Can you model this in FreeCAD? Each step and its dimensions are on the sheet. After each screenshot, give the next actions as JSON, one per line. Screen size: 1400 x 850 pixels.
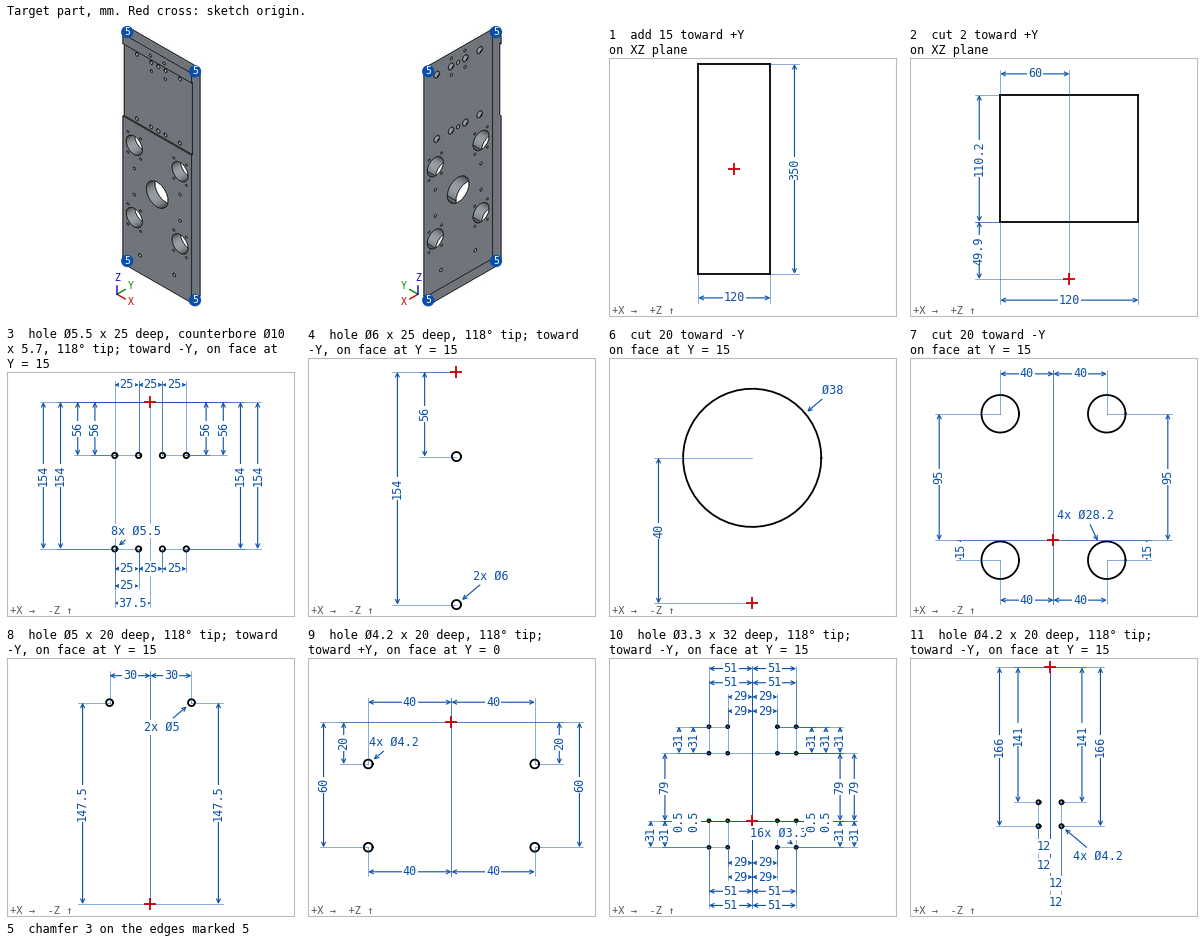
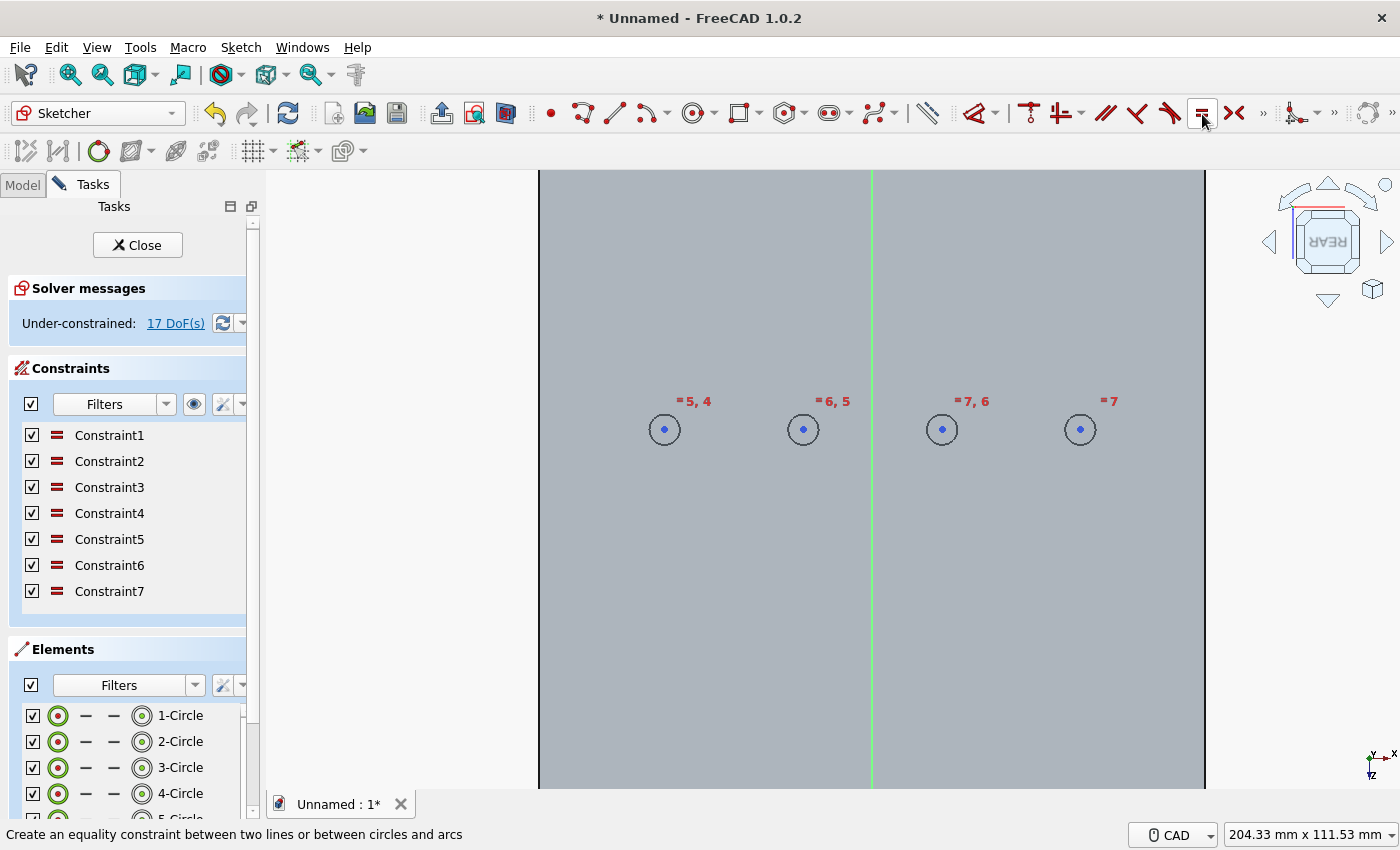
{"action": "scroll", "coordinate": [676, 419], "scroll_direction": "down", "scroll_amount": 4}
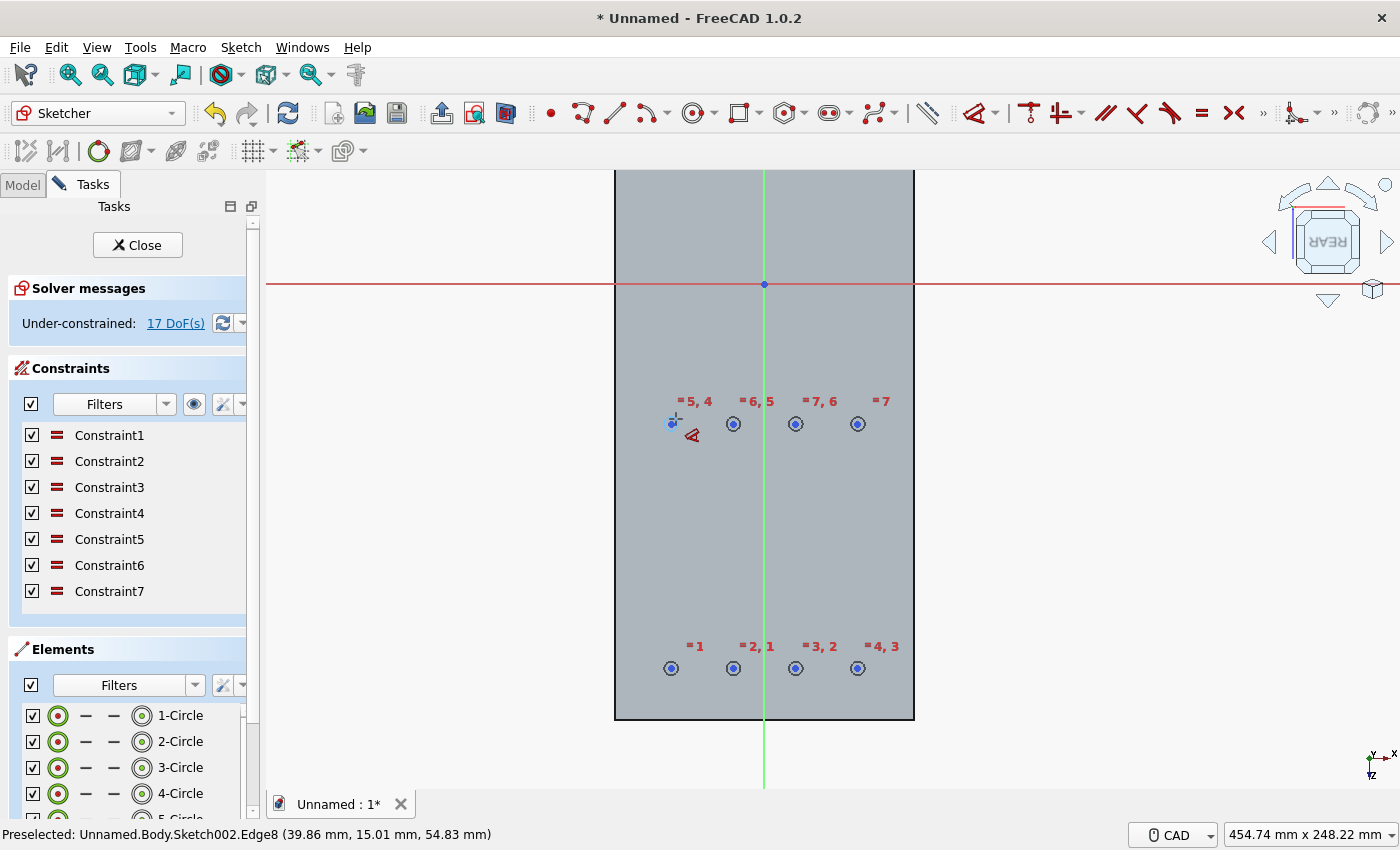
{"action": "scroll", "coordinate": [676, 664], "scroll_direction": "up", "scroll_amount": 6}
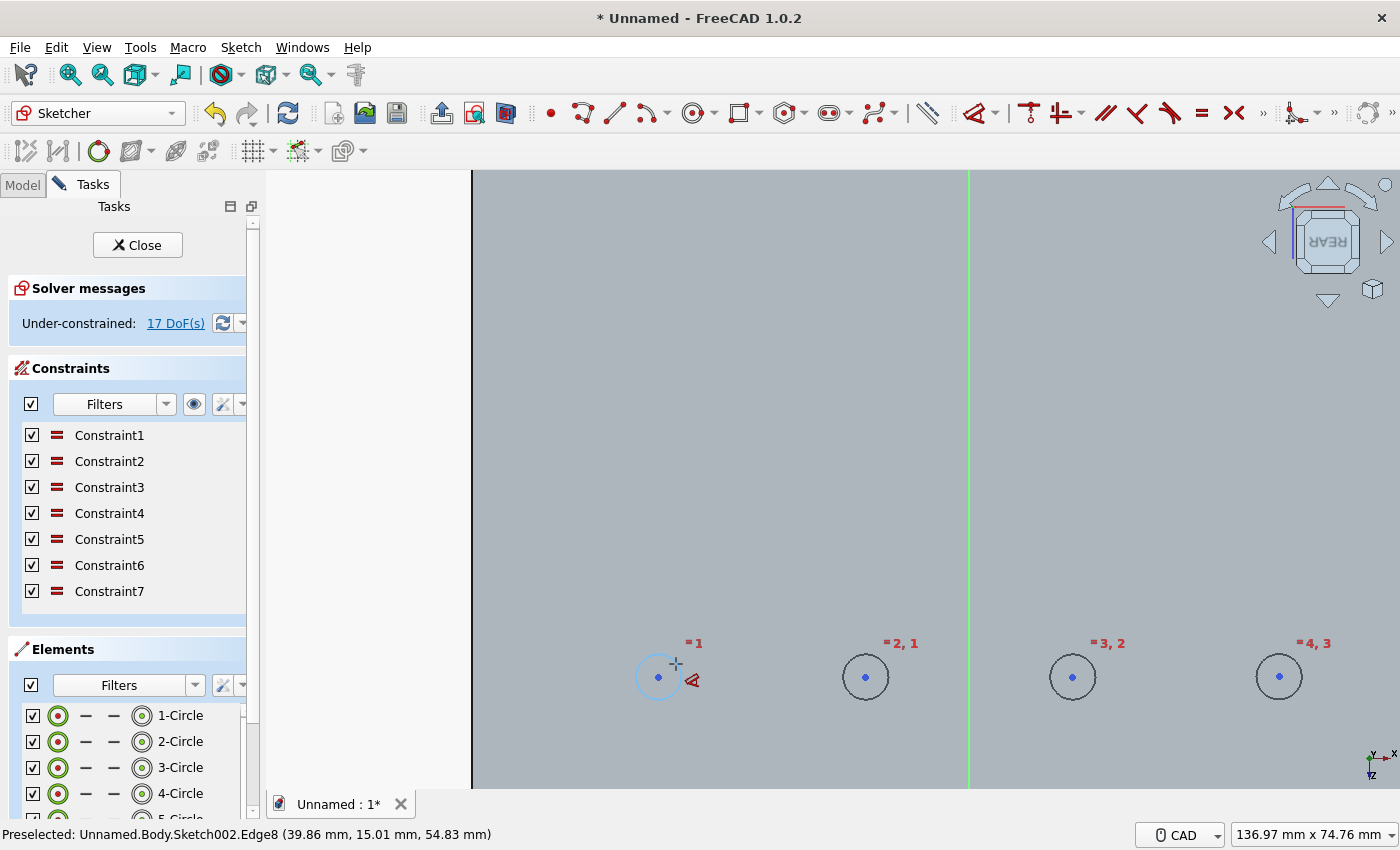
{"action": "left_click", "coordinate": [675, 661]}
{"action": "left_click", "coordinate": [698, 638]}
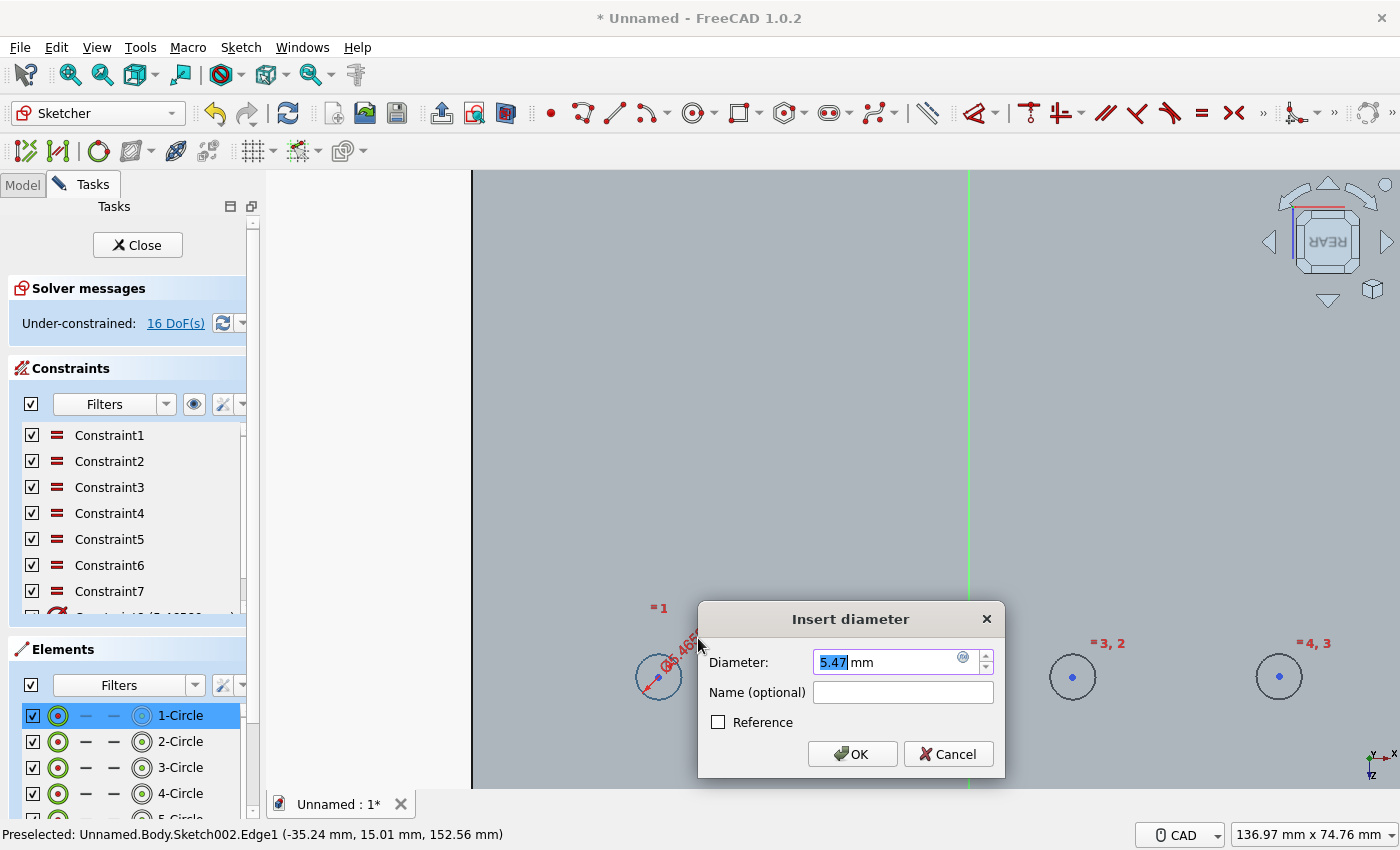
{"action": "type", "text": "5.5"}
{"action": "key", "text": "Return"}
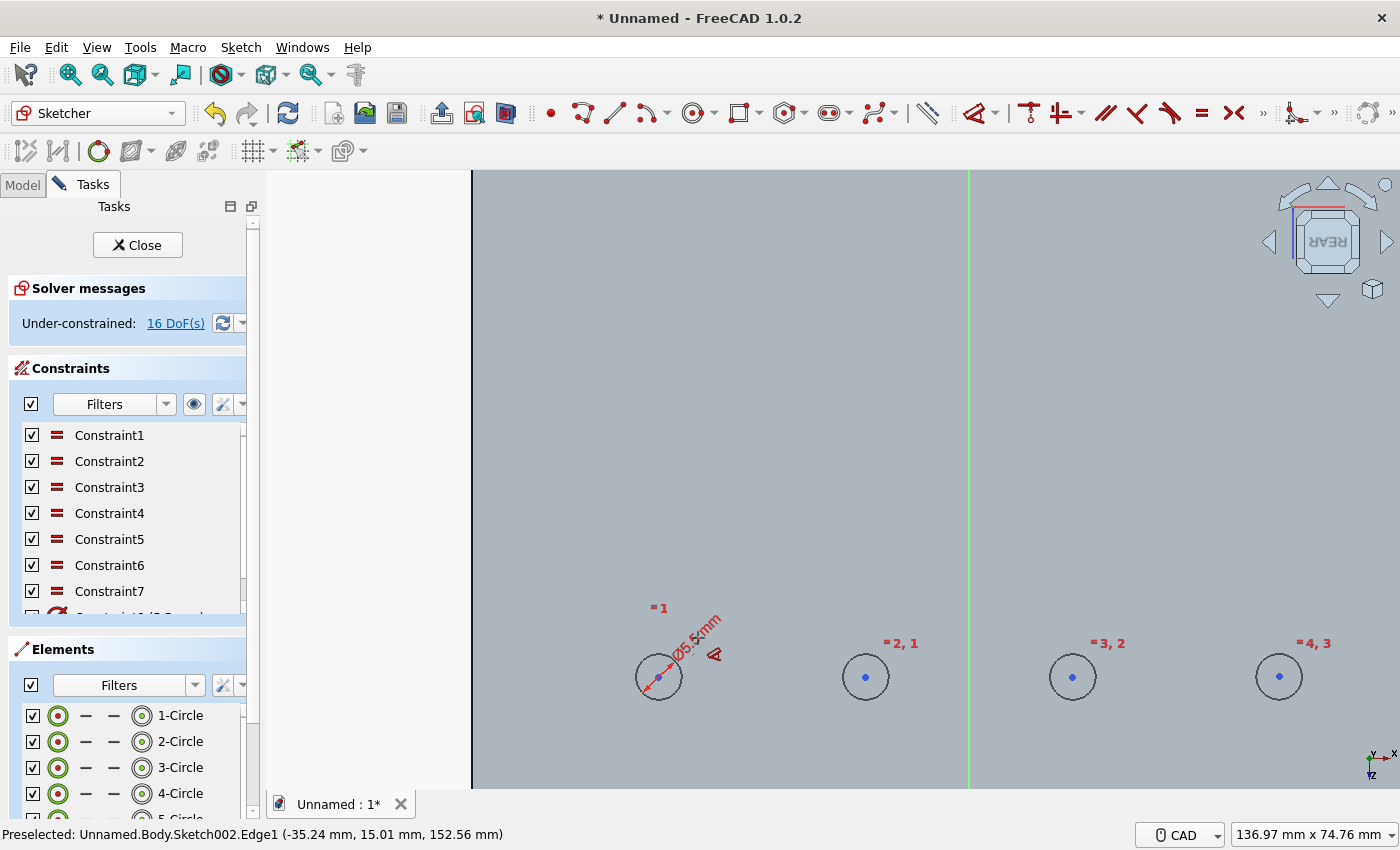
{"action": "scroll", "coordinate": [676, 665], "scroll_direction": "down", "scroll_amount": 6}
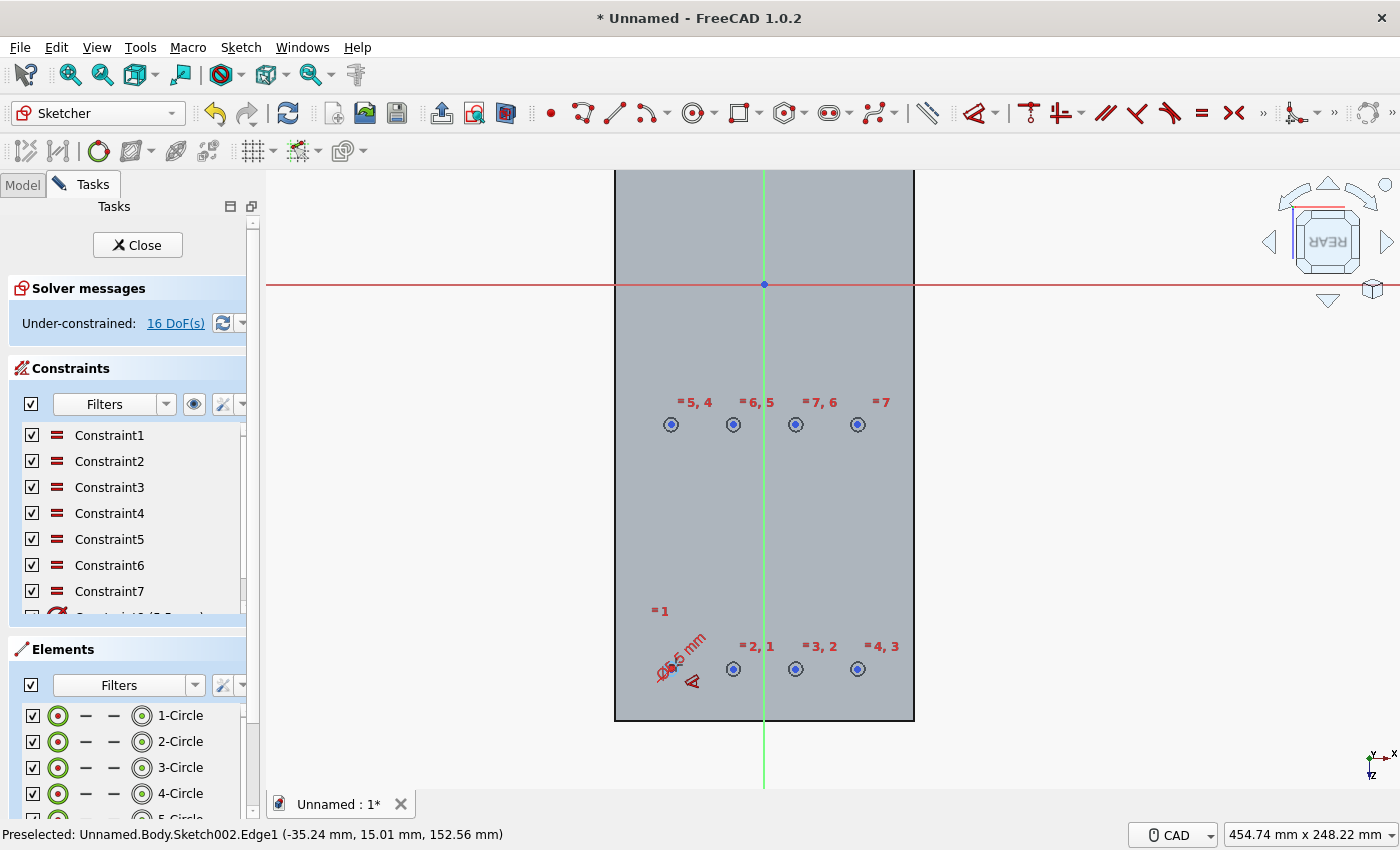
{"action": "left_click", "coordinate": [671, 425]}
{"action": "left_click", "coordinate": [637, 355]}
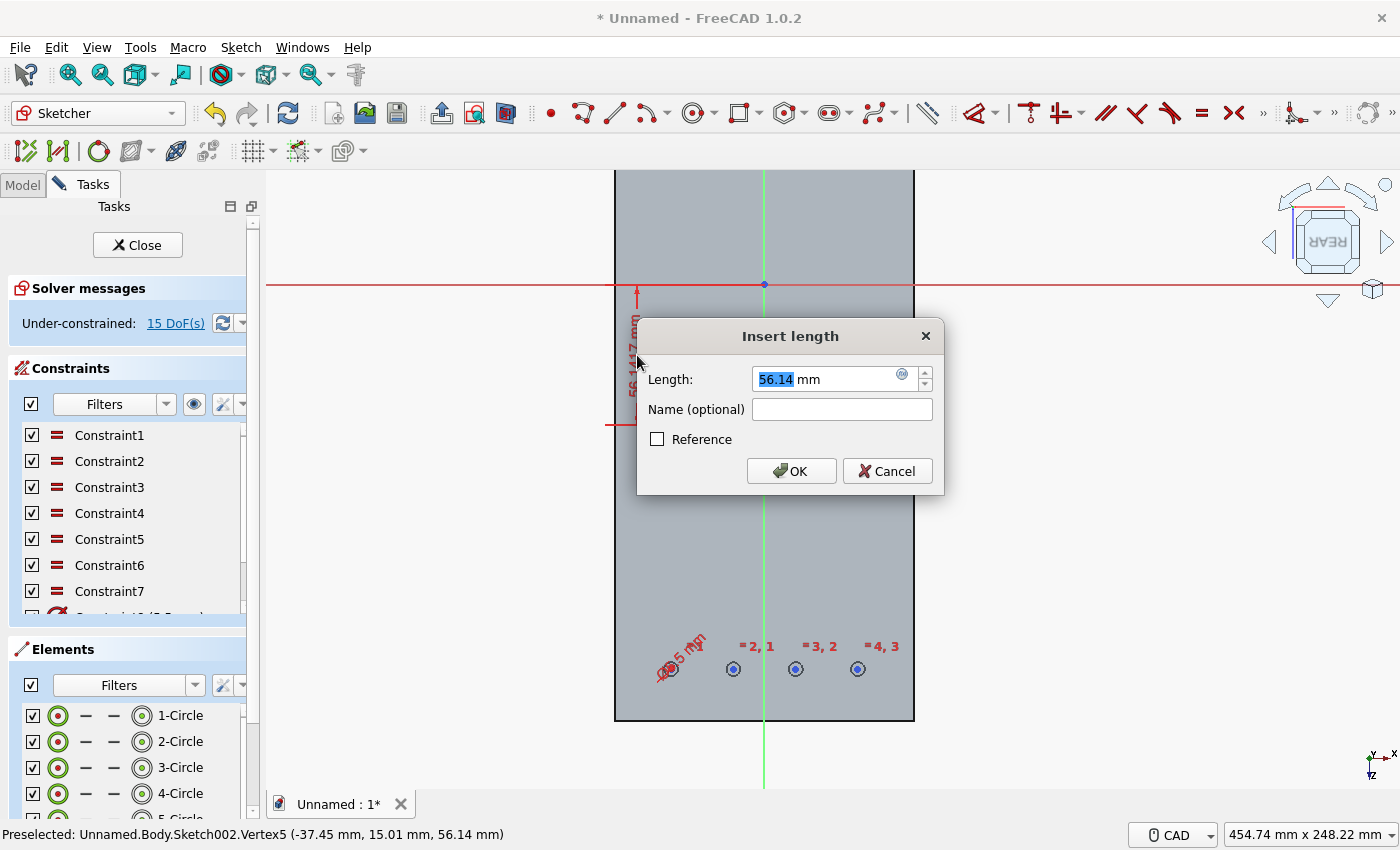
{"action": "type", "text": "56"}
{"action": "key", "text": "Return"}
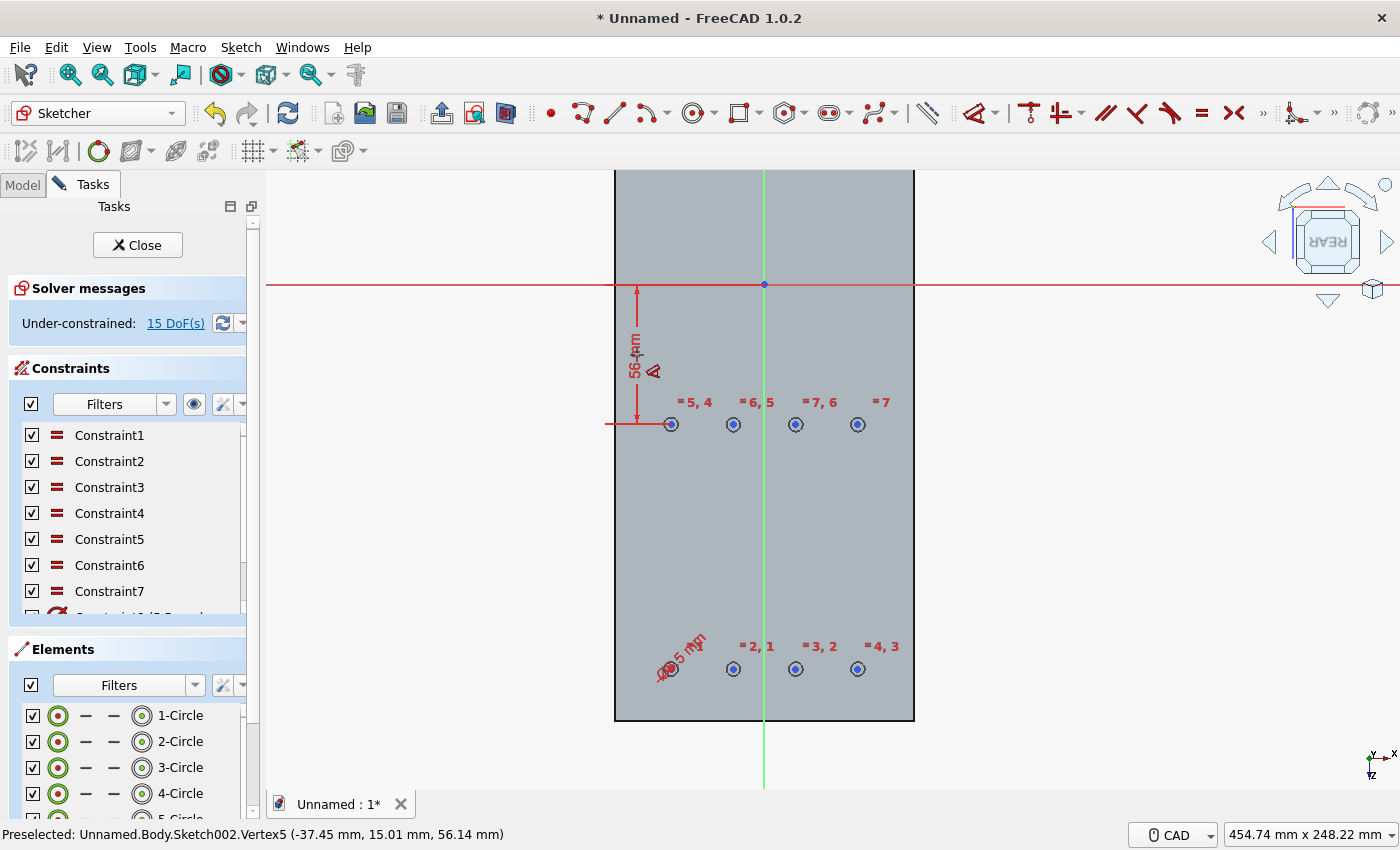
{"action": "left_click", "coordinate": [733, 425]}
{"action": "left_click", "coordinate": [699, 323]}